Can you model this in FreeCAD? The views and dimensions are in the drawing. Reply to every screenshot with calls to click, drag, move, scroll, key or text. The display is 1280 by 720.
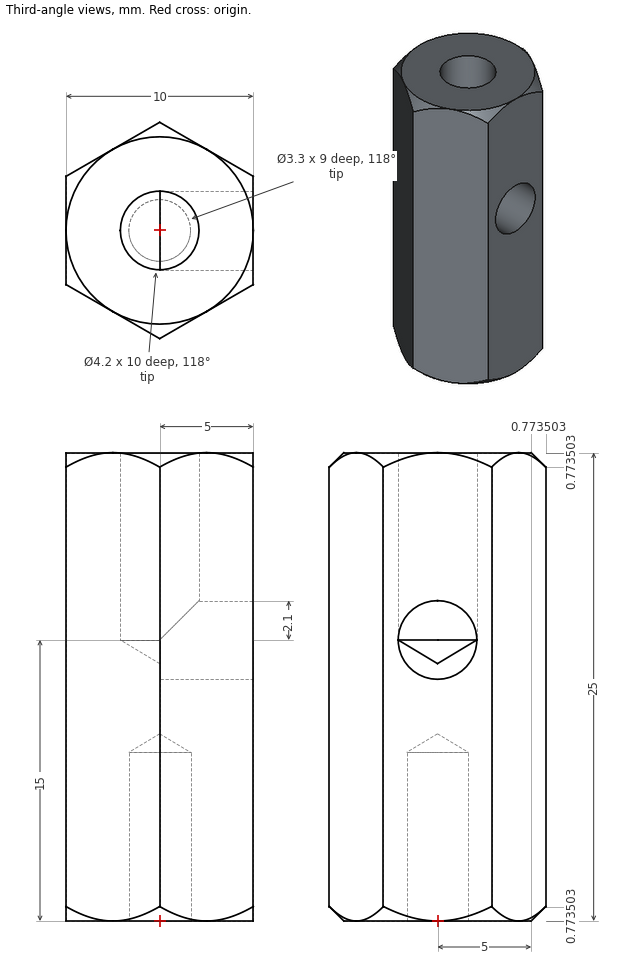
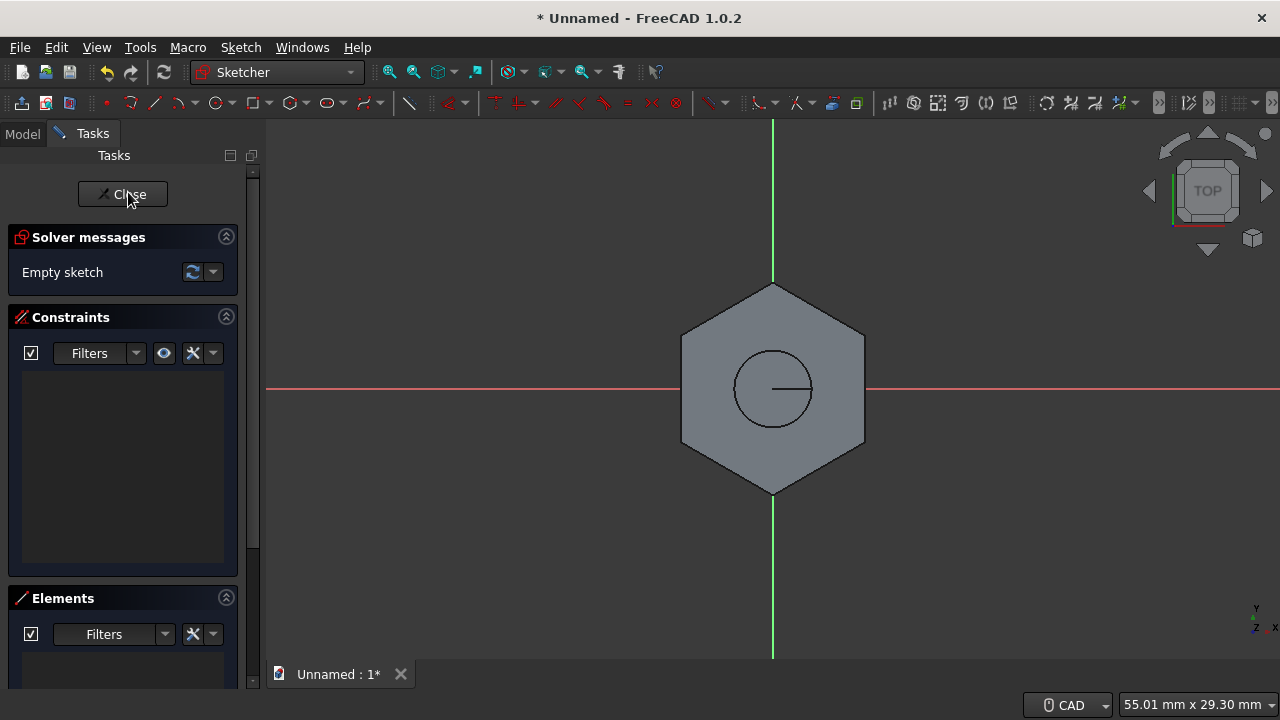
key(q)
key(s)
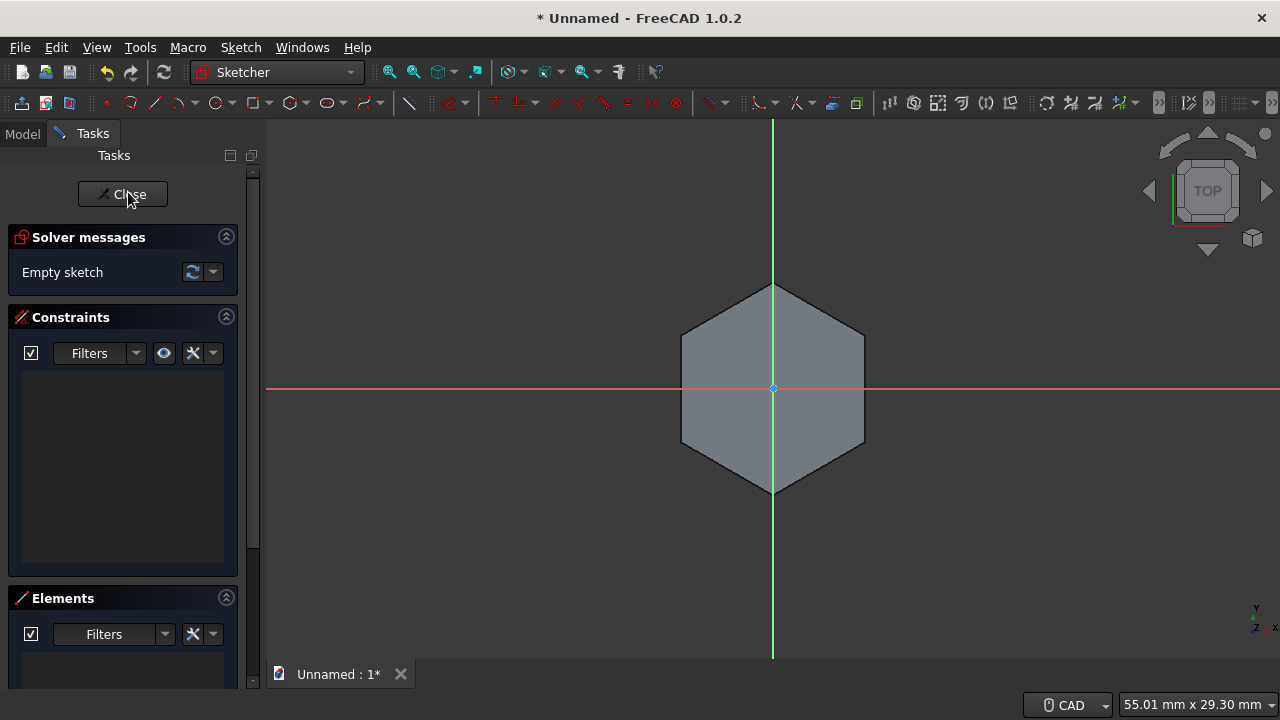
scroll(787, 389, up, 9)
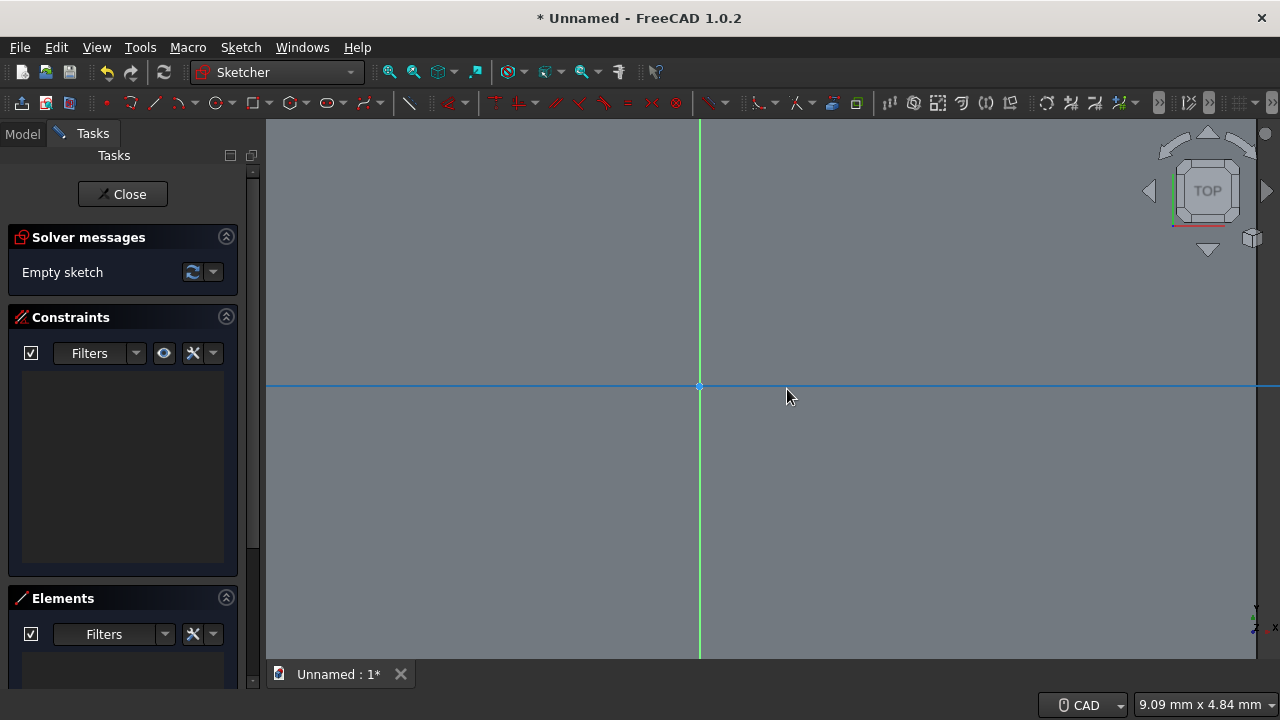
click(216, 104)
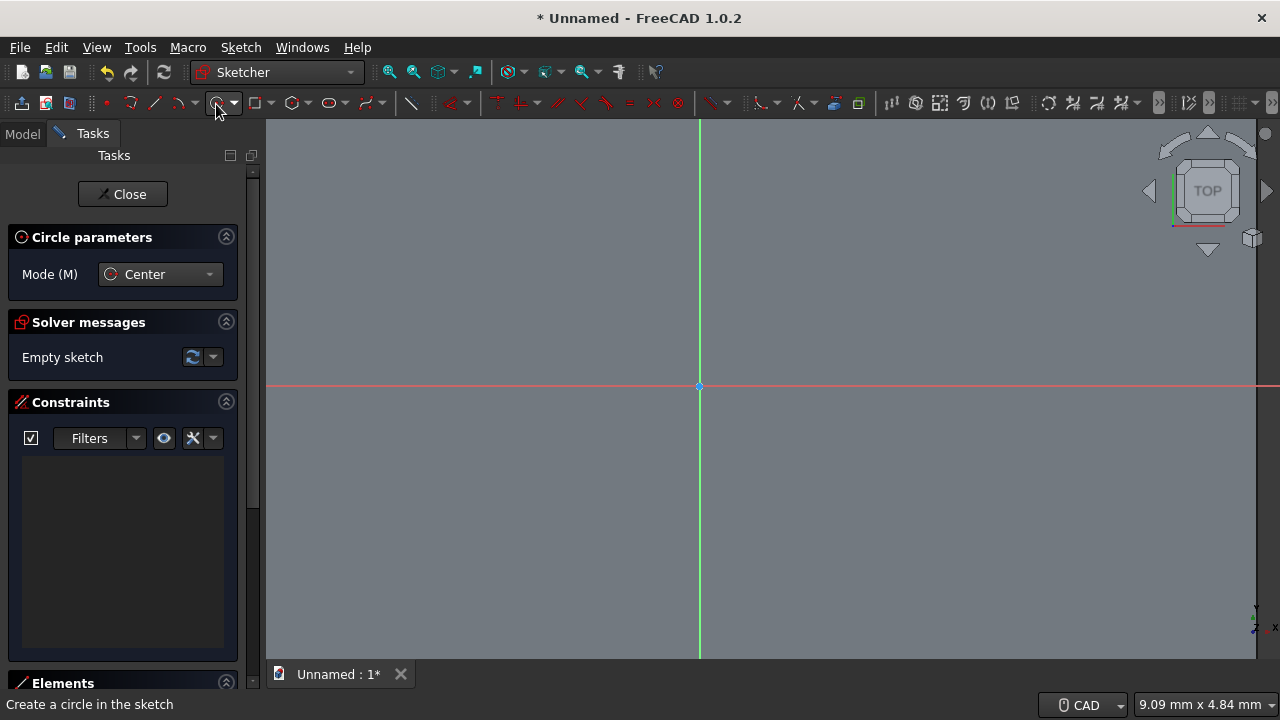
click(700, 386)
move(830, 256)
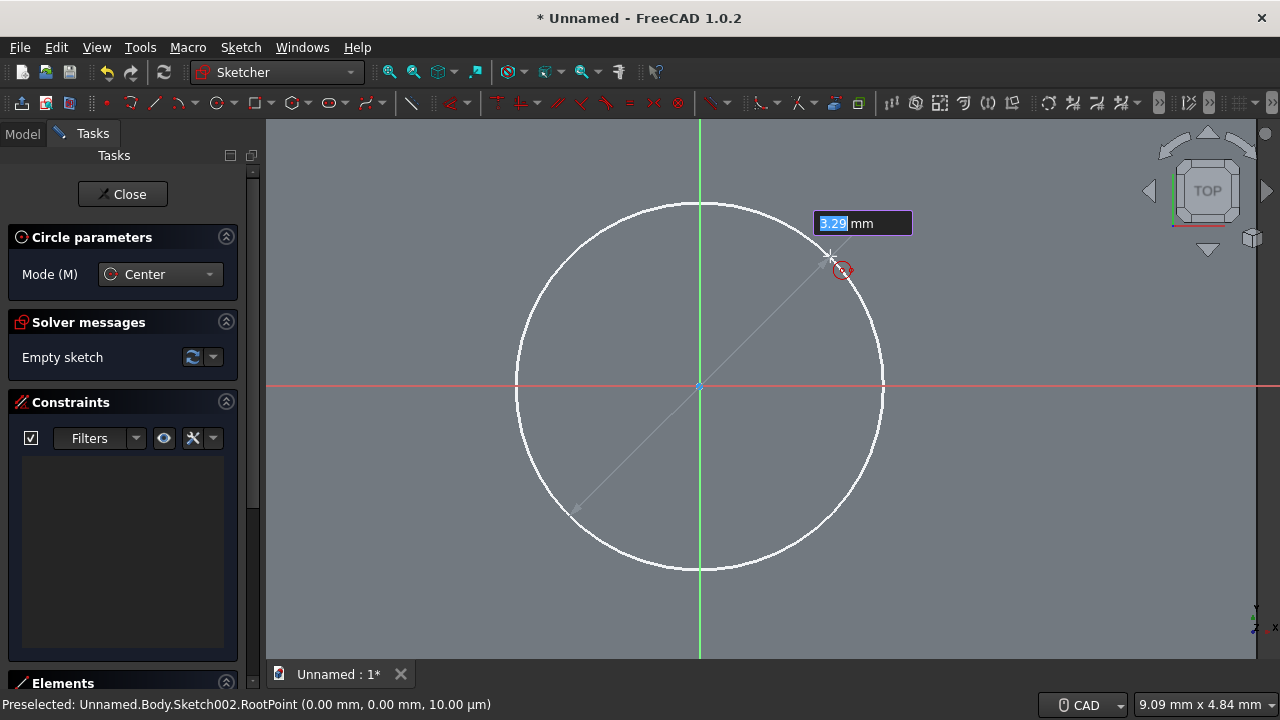
text(3.3)
key(Return)
key(Escape)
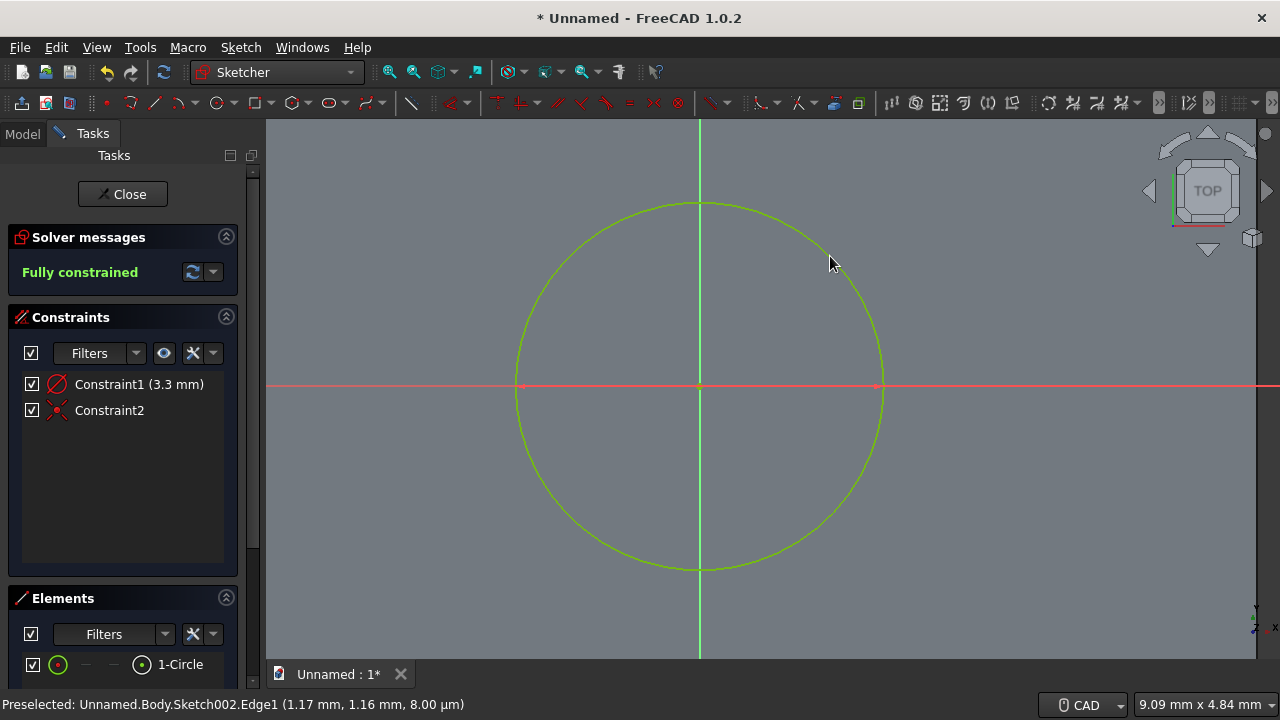
click(123, 194)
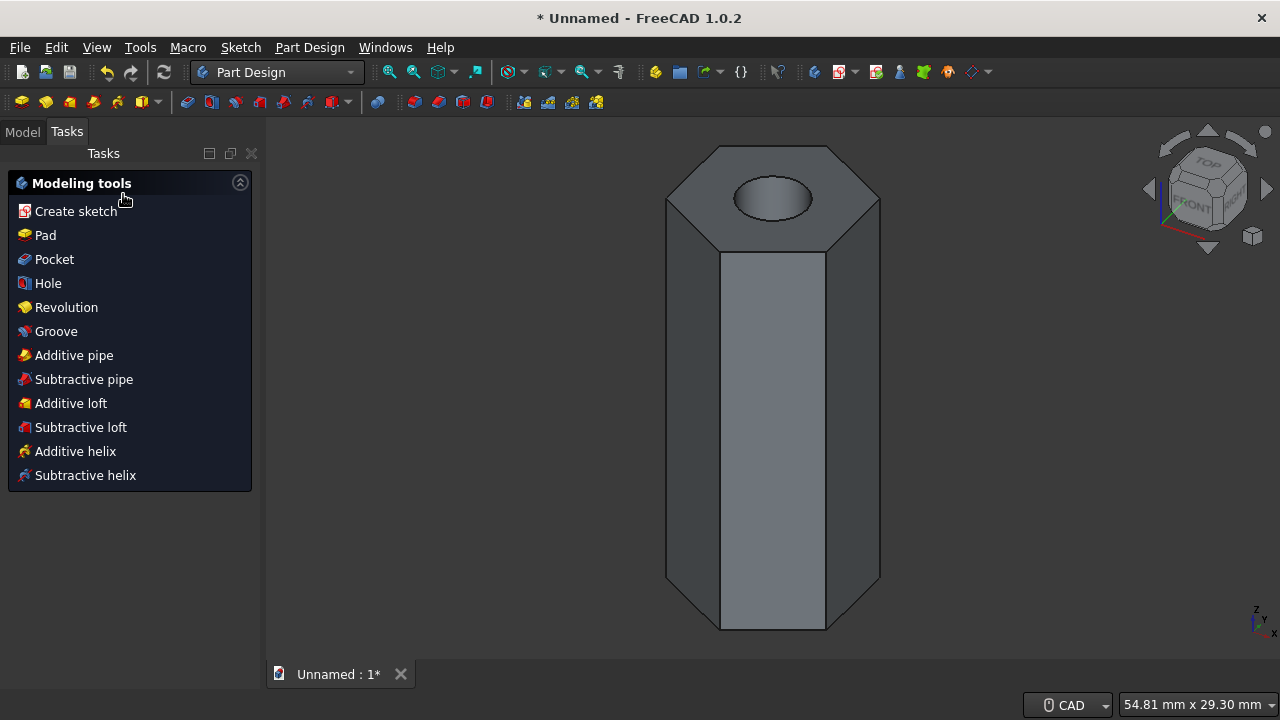
click(212, 102)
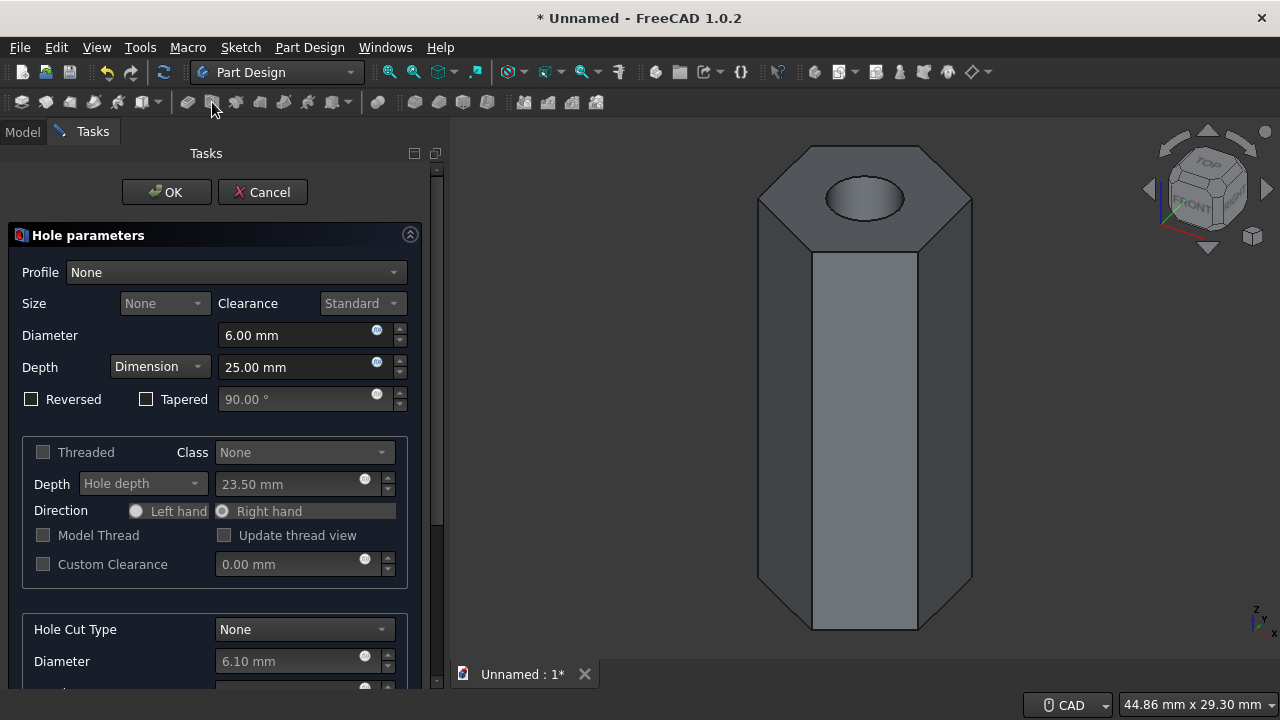
triple_click(305, 335)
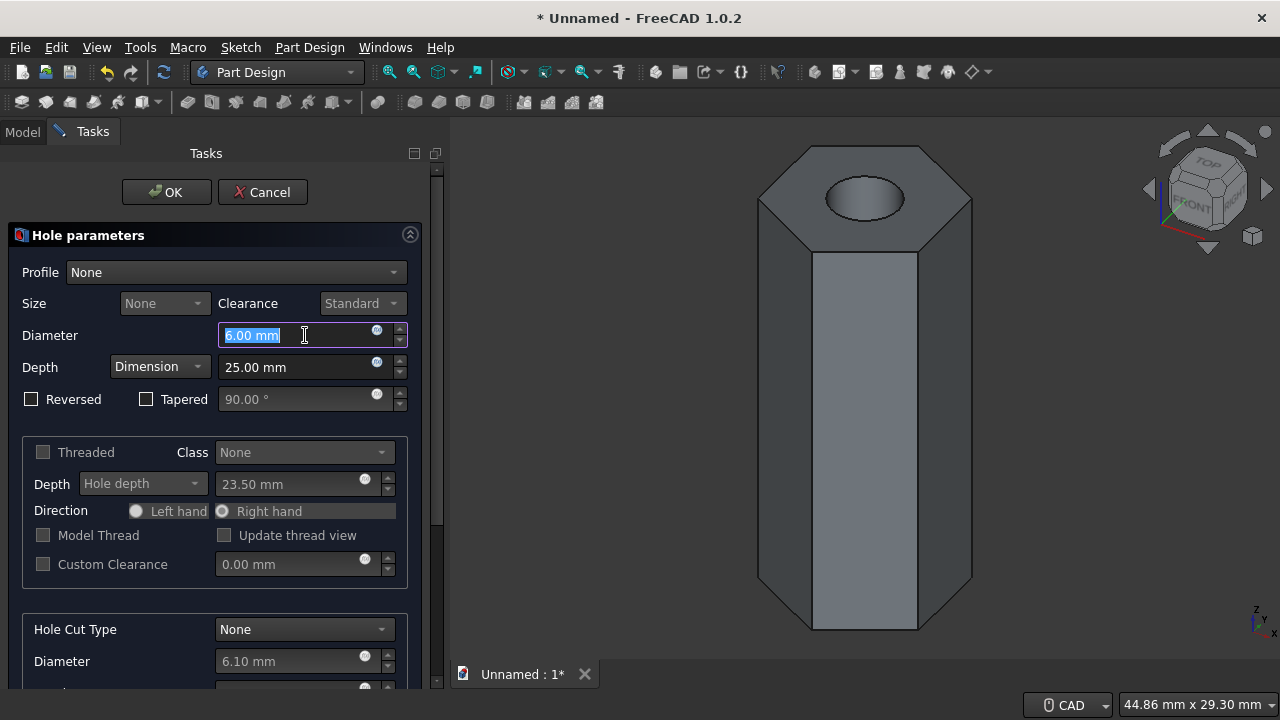
text(3.3)
key(Tab)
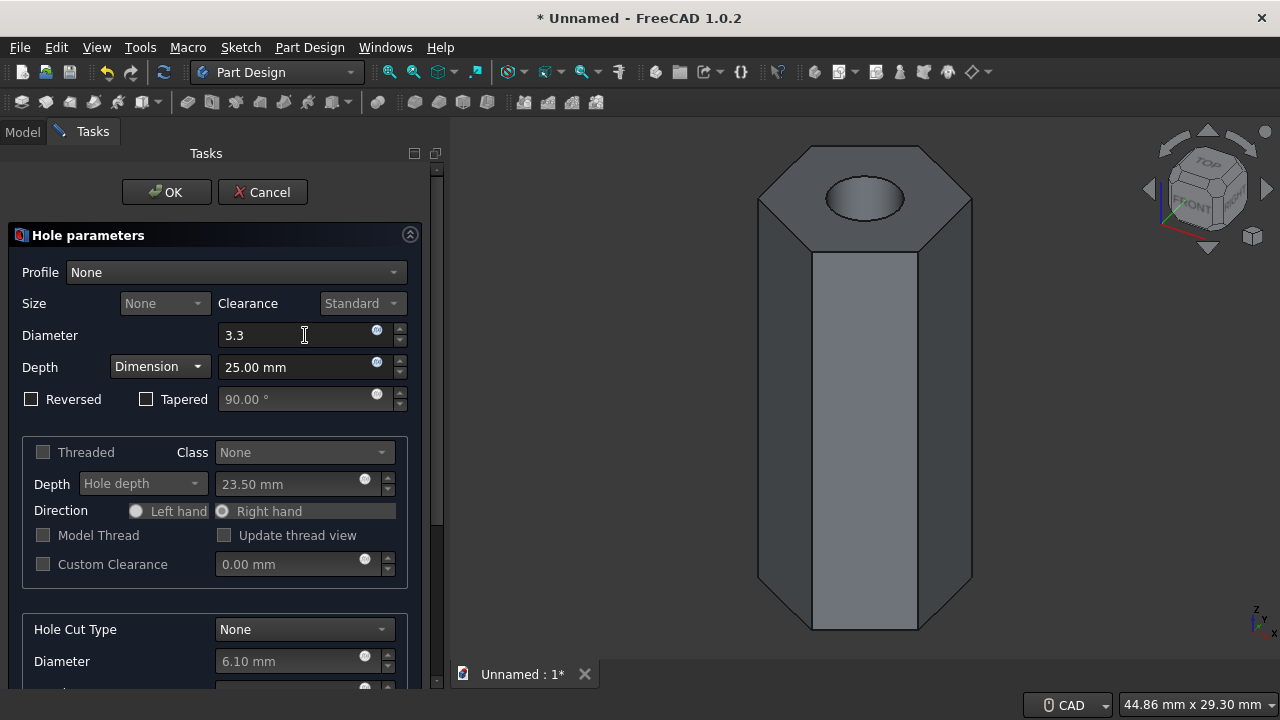
triple_click(305, 367)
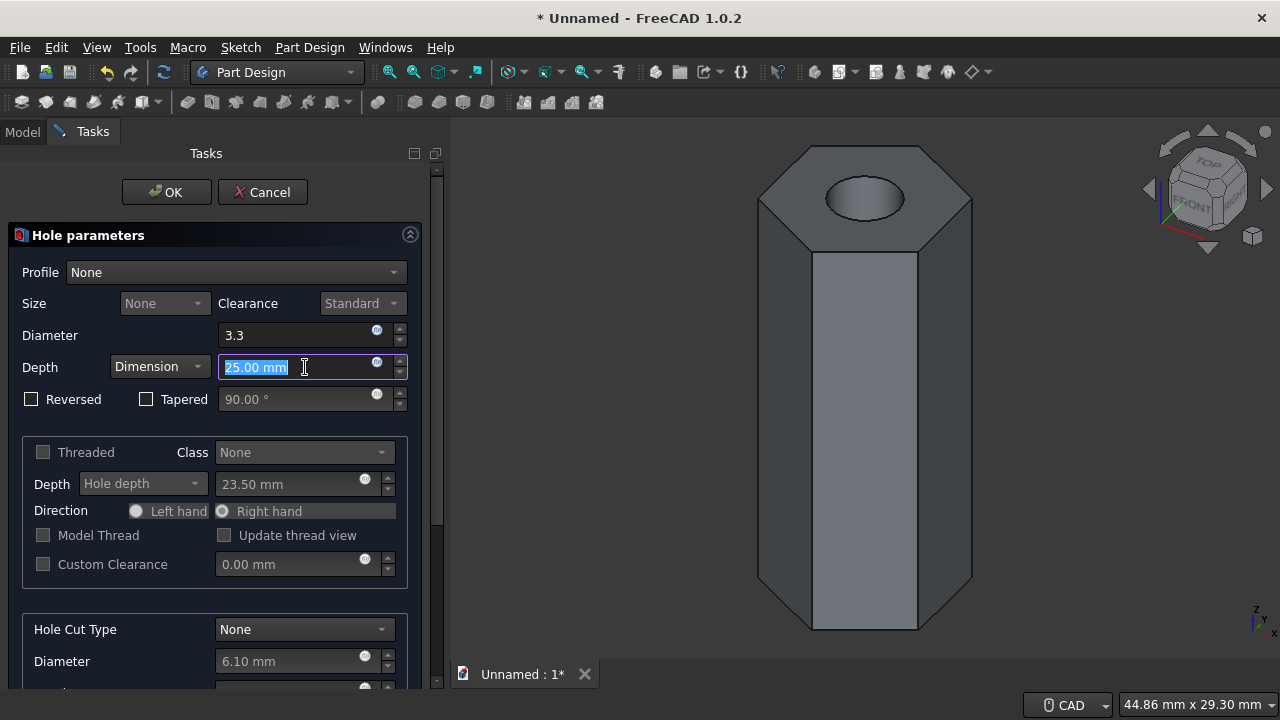
text(9)
key(Tab)